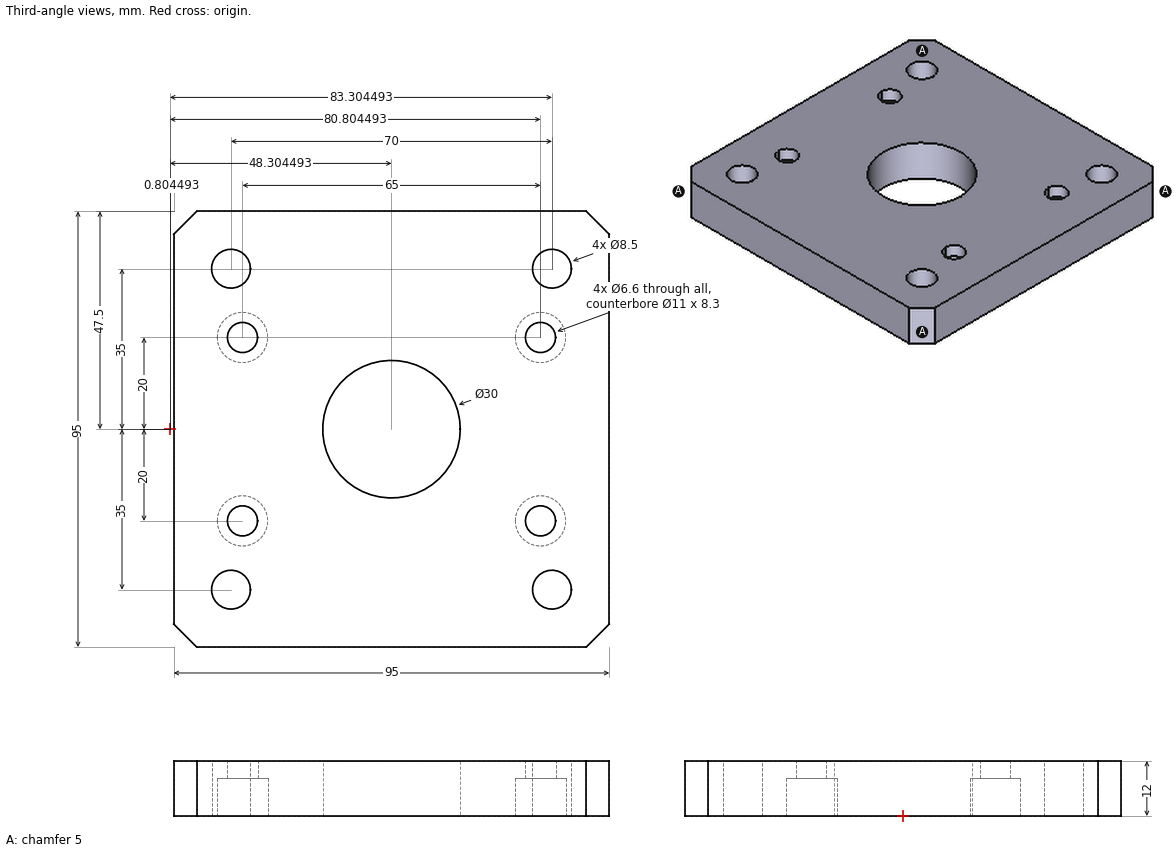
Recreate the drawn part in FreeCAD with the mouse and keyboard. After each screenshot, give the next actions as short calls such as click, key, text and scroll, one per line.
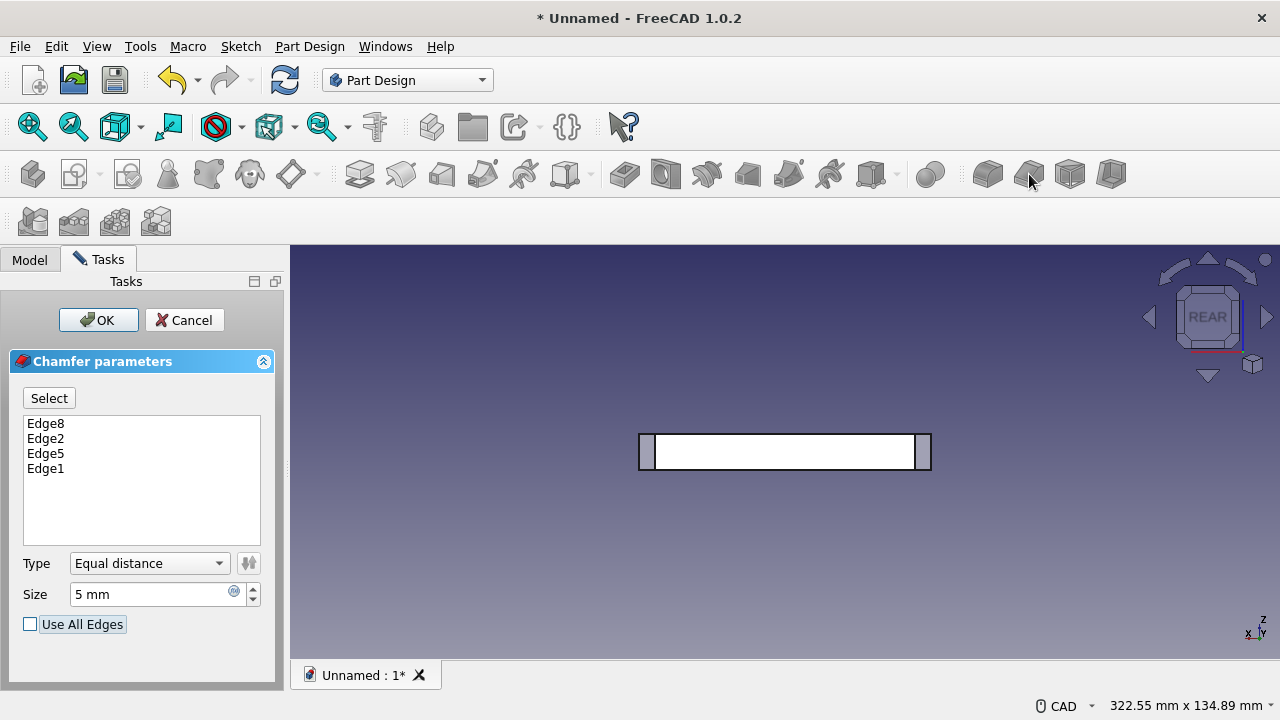
click(99, 320)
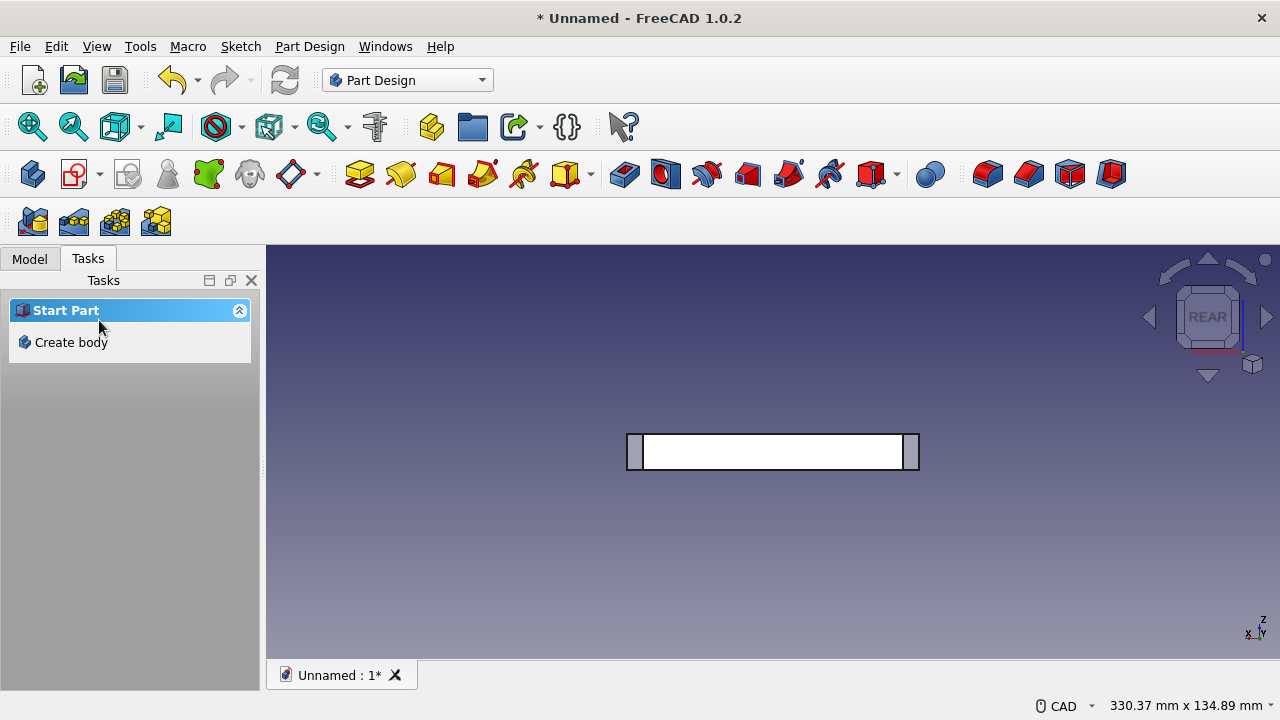
key(0)